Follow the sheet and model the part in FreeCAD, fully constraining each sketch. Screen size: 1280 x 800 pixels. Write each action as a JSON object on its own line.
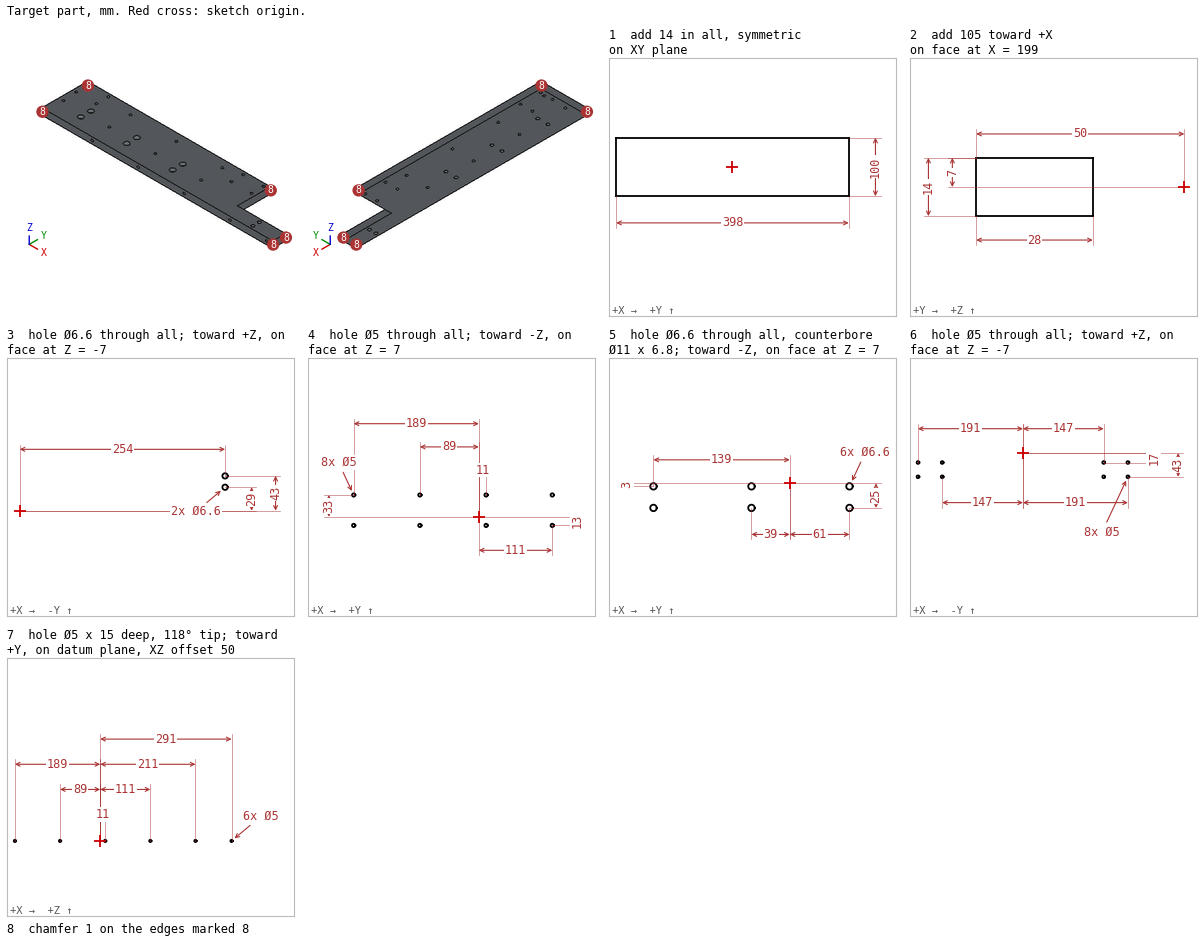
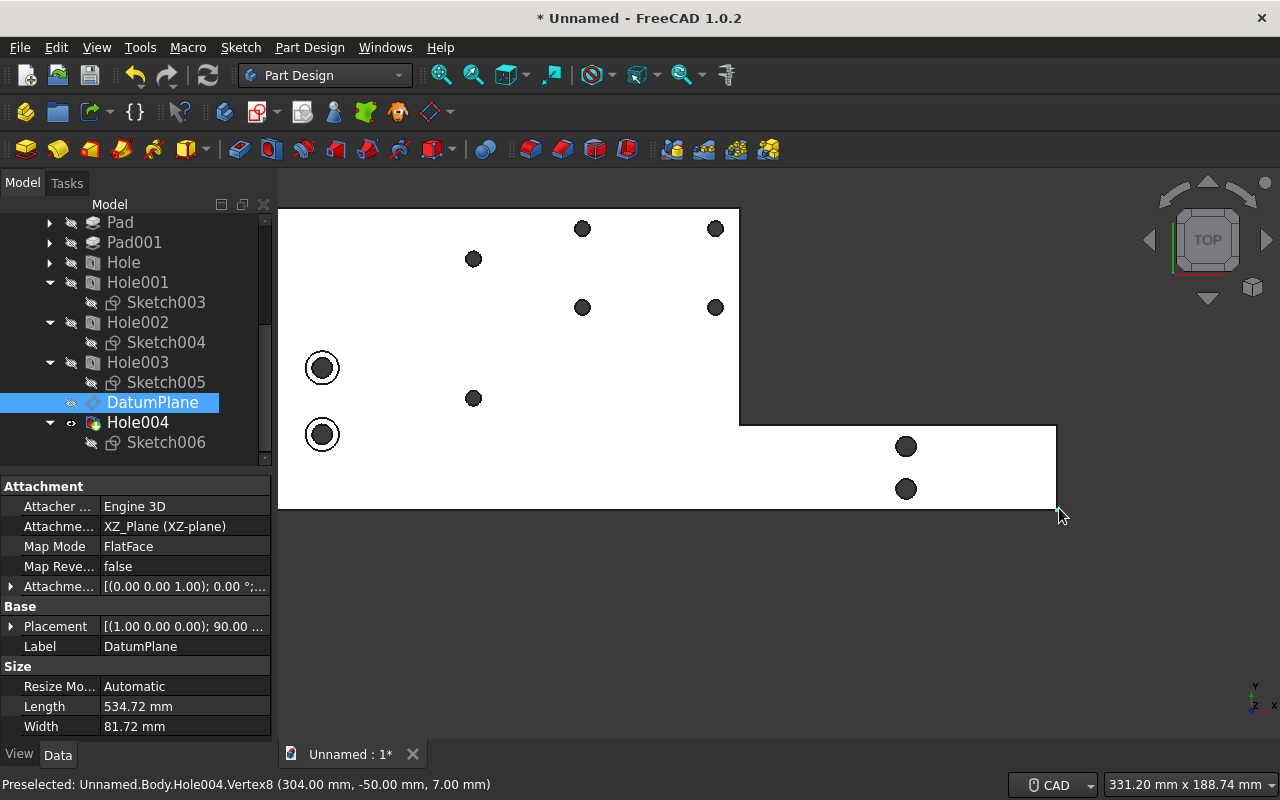
{"action": "key", "text": "v f"}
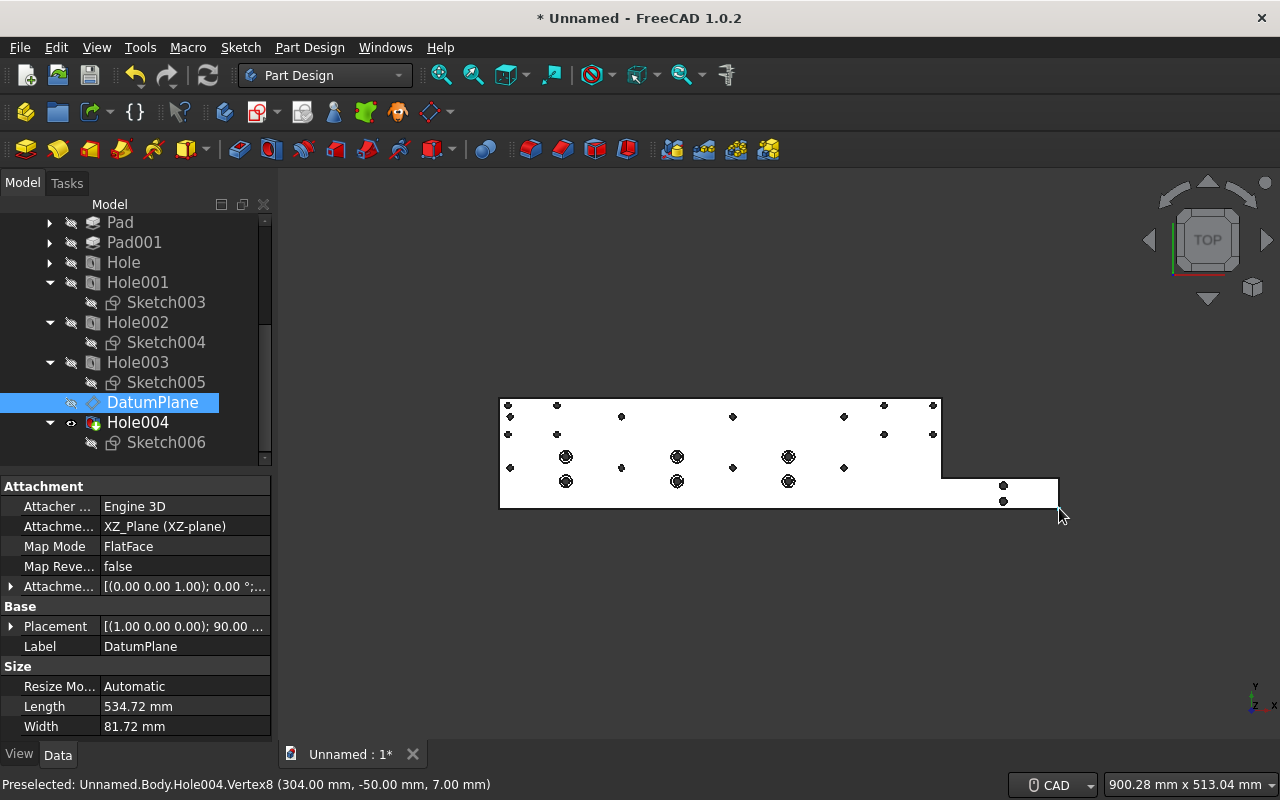
{"action": "key", "text": "0"}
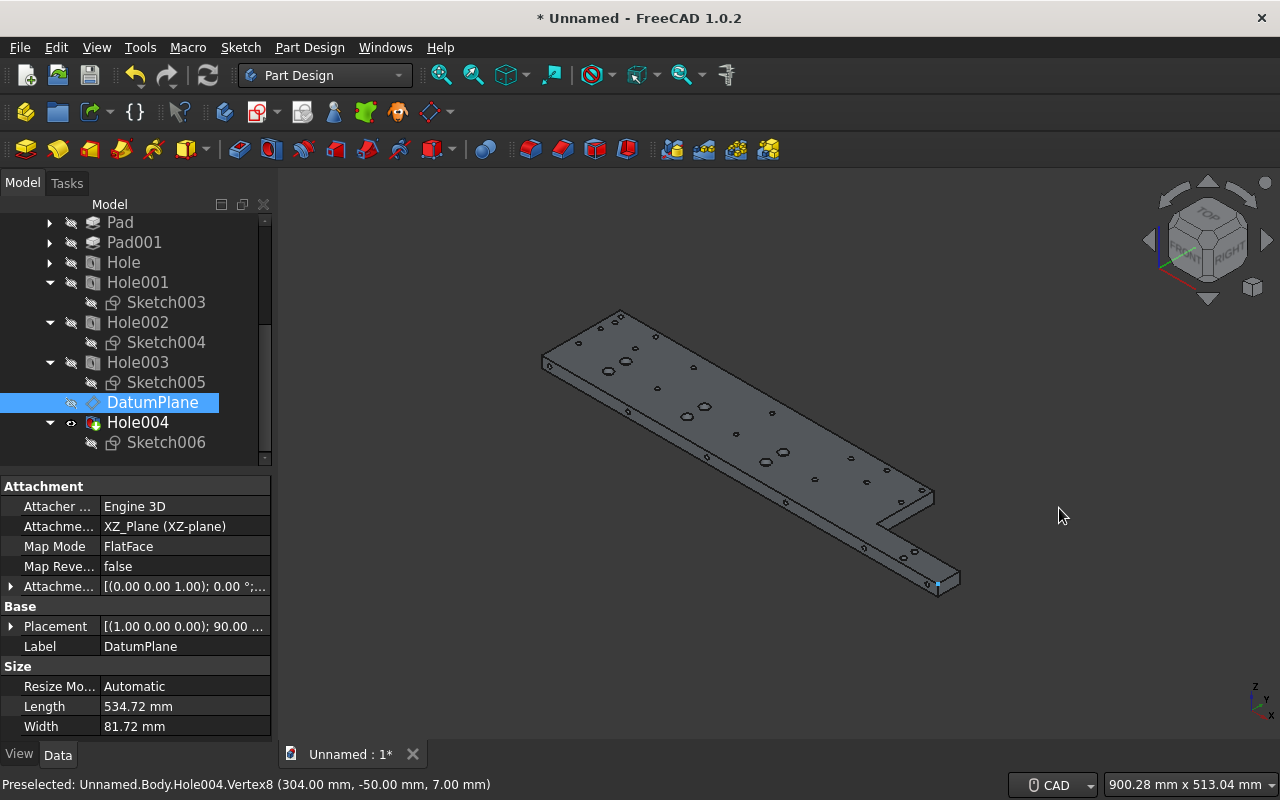
{"action": "left_click", "coordinate": [938, 591]}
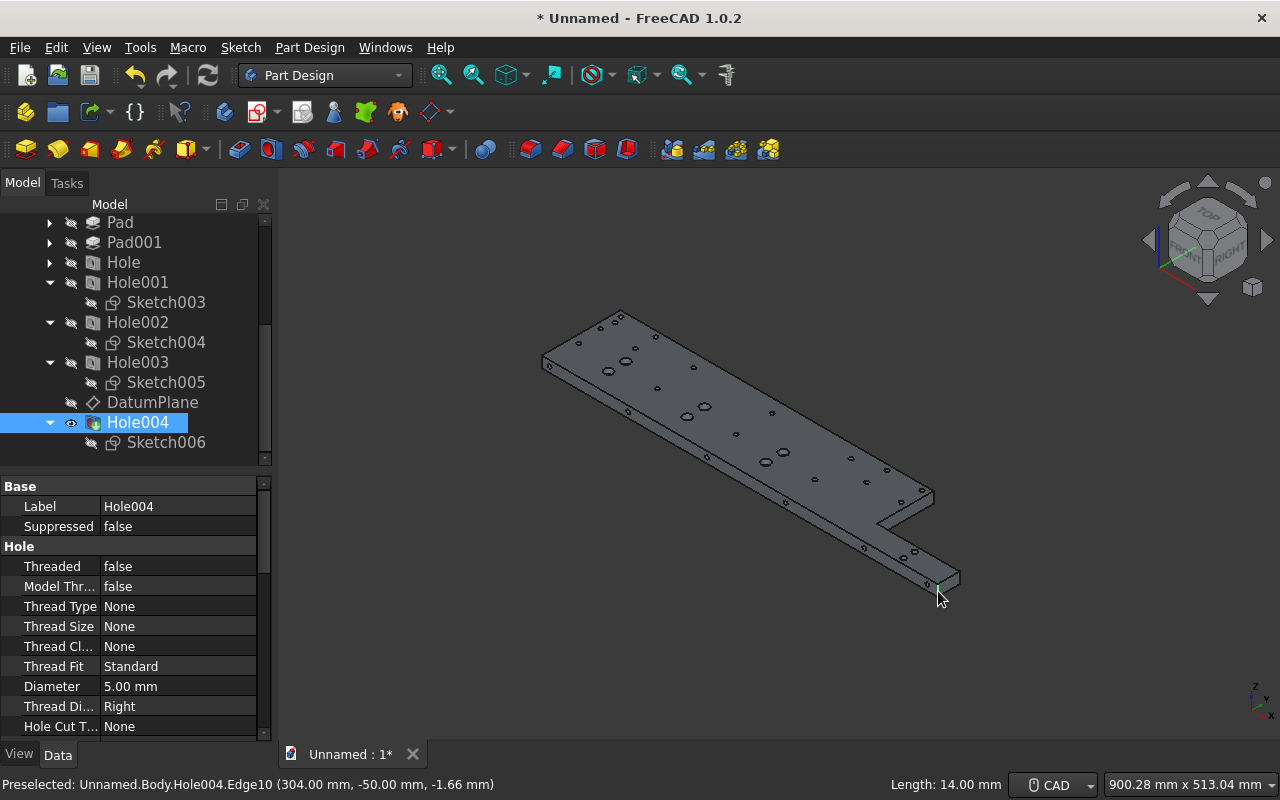
{"action": "scroll", "coordinate": [960, 577], "scroll_direction": "up", "scroll_amount": 5}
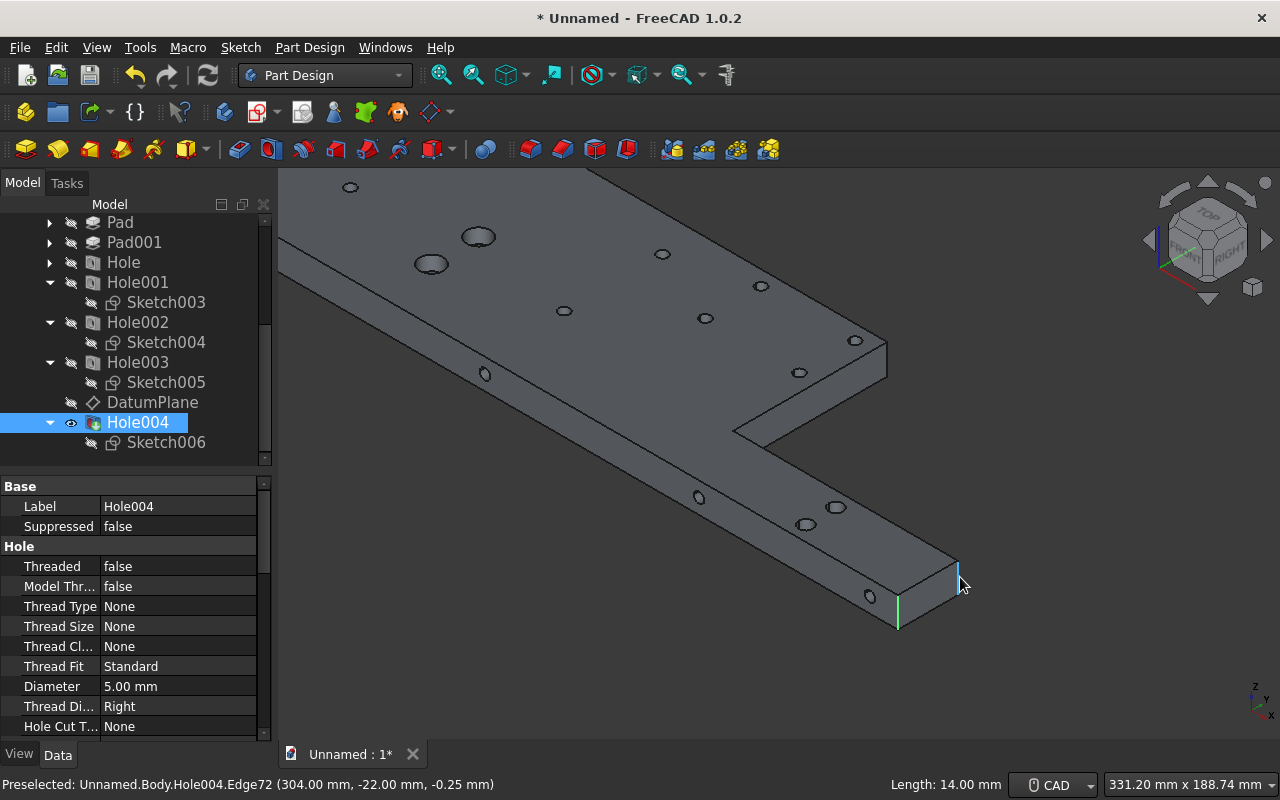
{"action": "key", "text": "v f"}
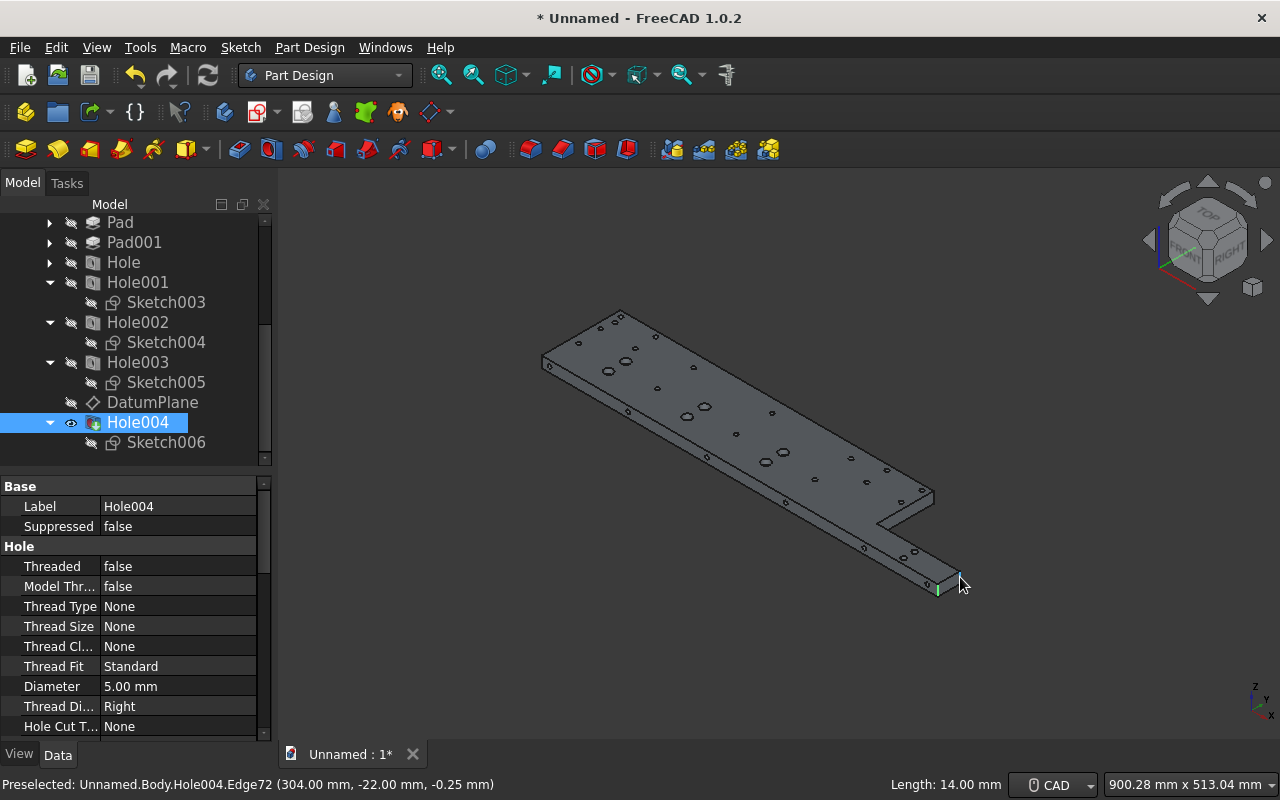
{"action": "key", "text": "2"}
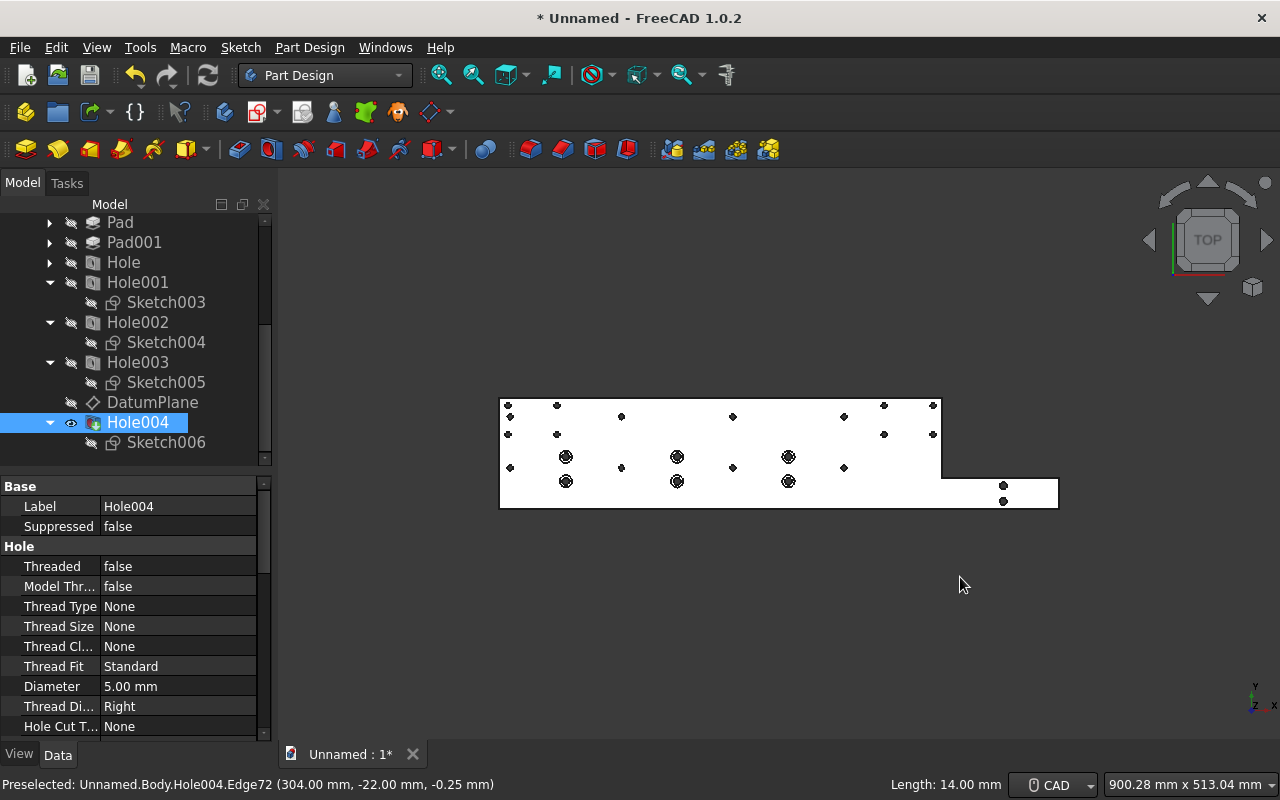
{"action": "scroll", "coordinate": [1059, 477], "scroll_direction": "up", "scroll_amount": 5}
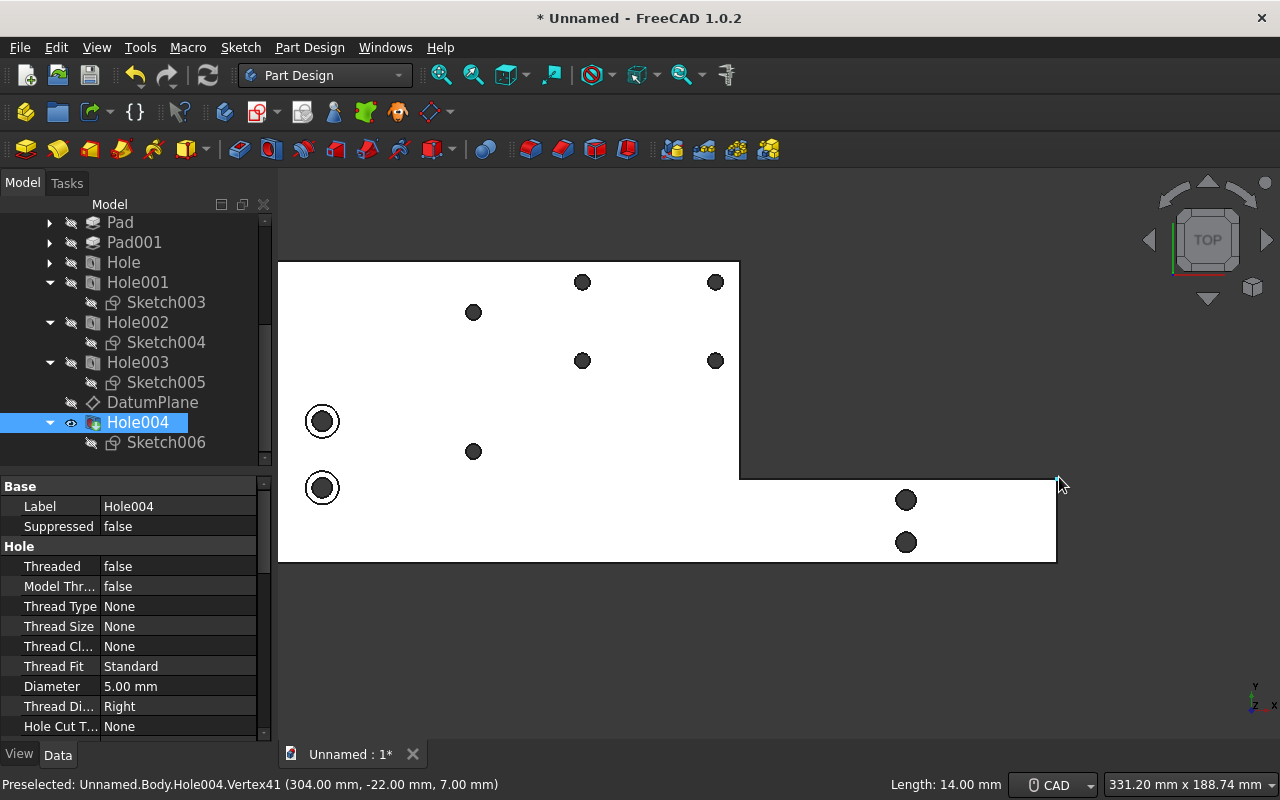
{"action": "key", "text": "v f"}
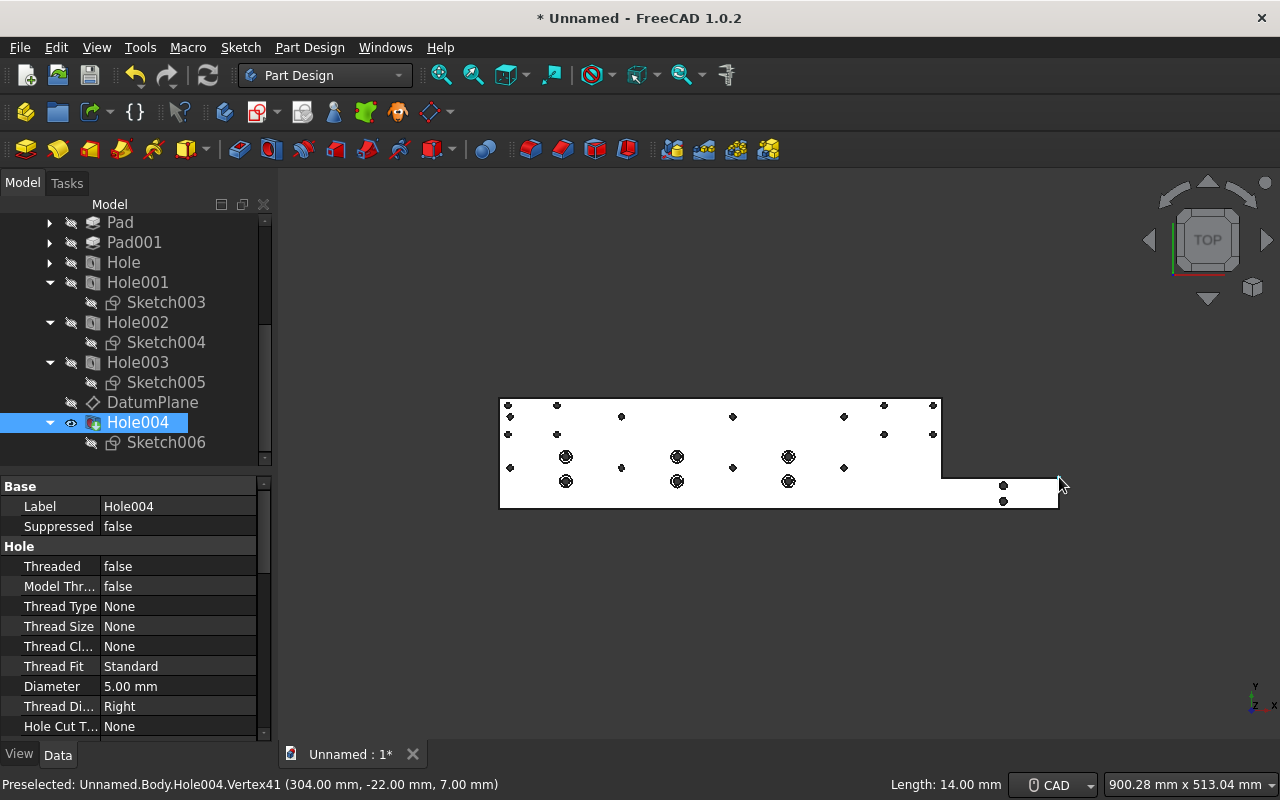
{"action": "key", "text": "1"}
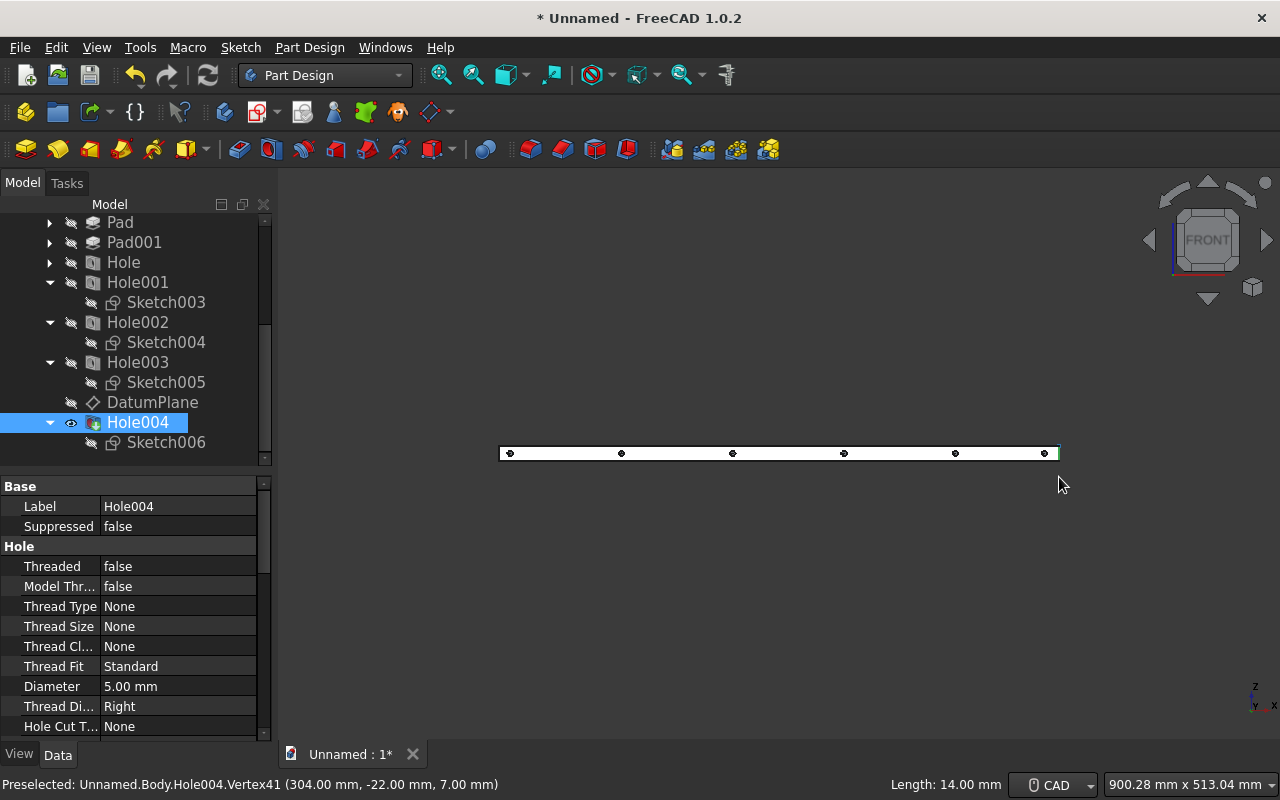
{"action": "left_click", "coordinate": [499, 452], "text": "ctrl"}